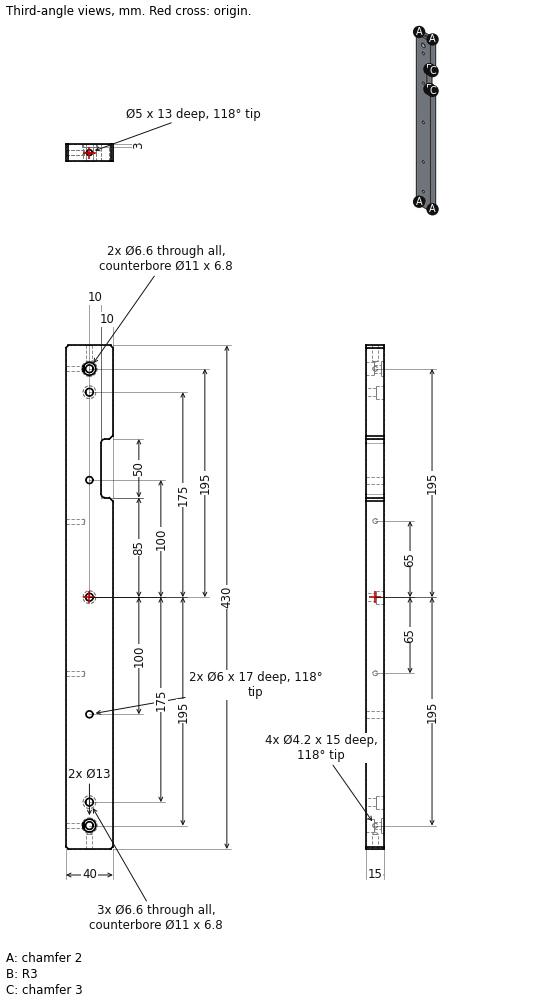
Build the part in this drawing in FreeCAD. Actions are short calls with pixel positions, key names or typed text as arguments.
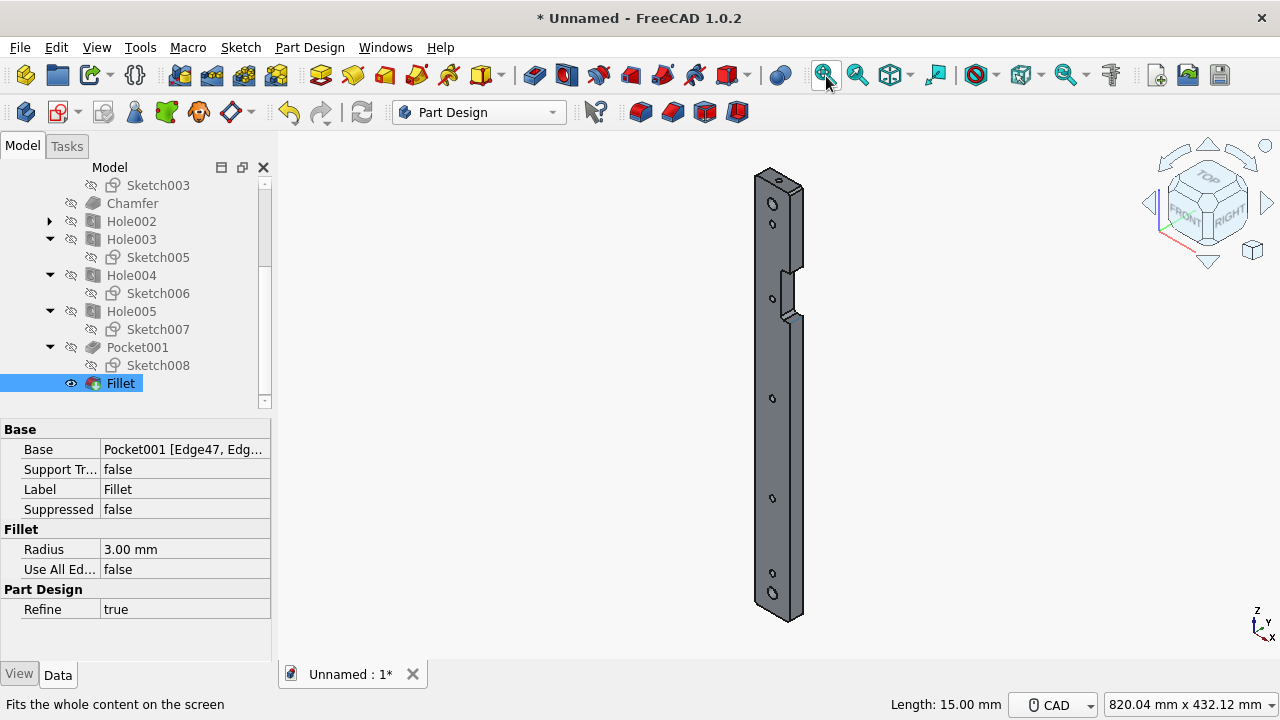
key(2)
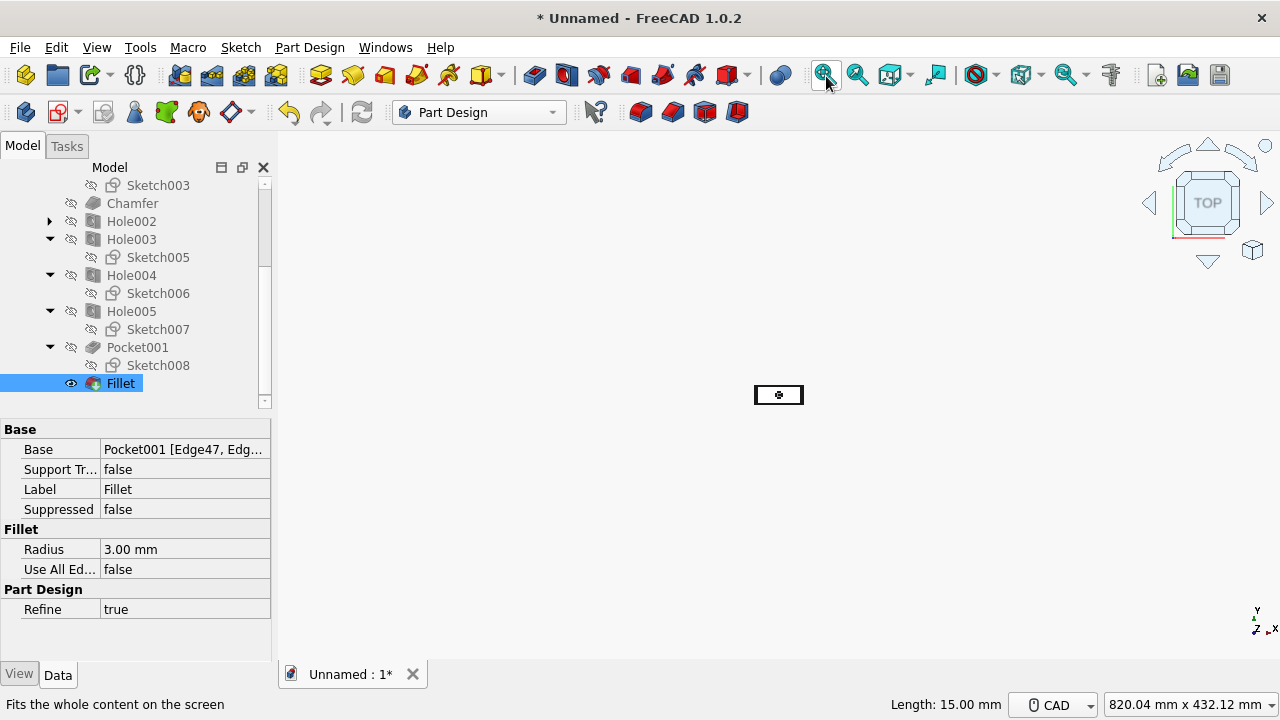
click(826, 76)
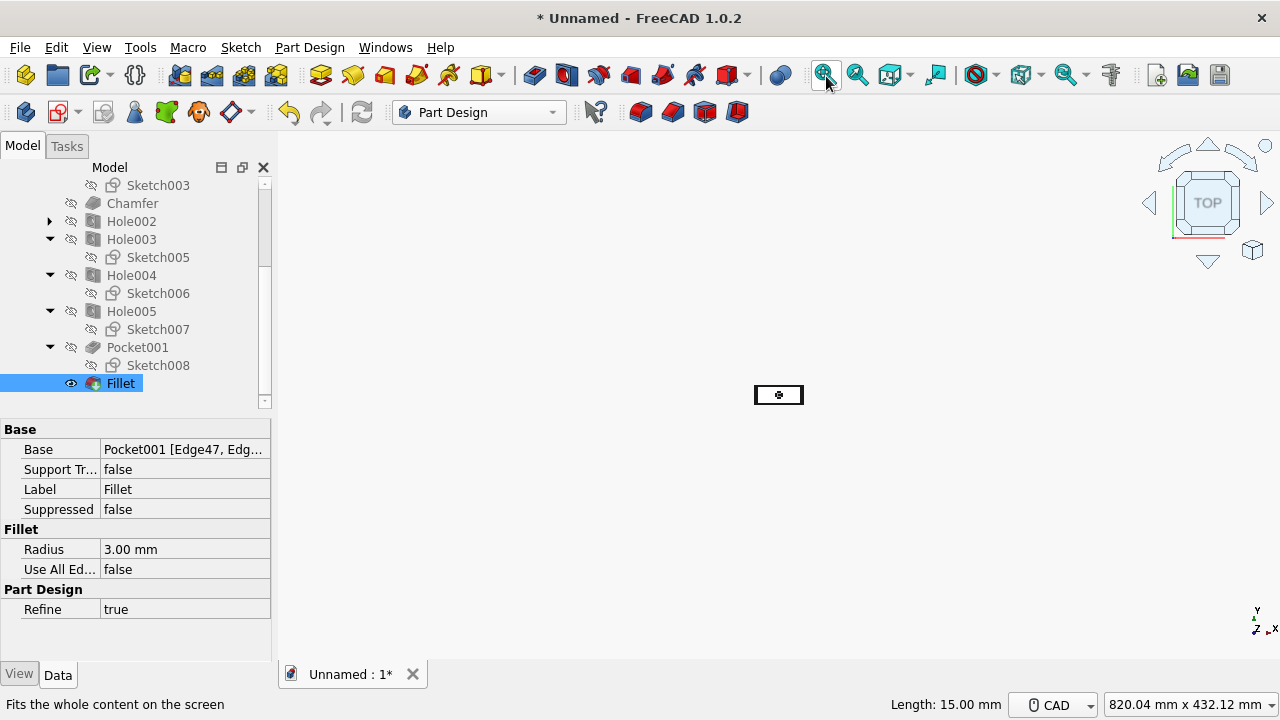
scroll(803, 394, up, 4)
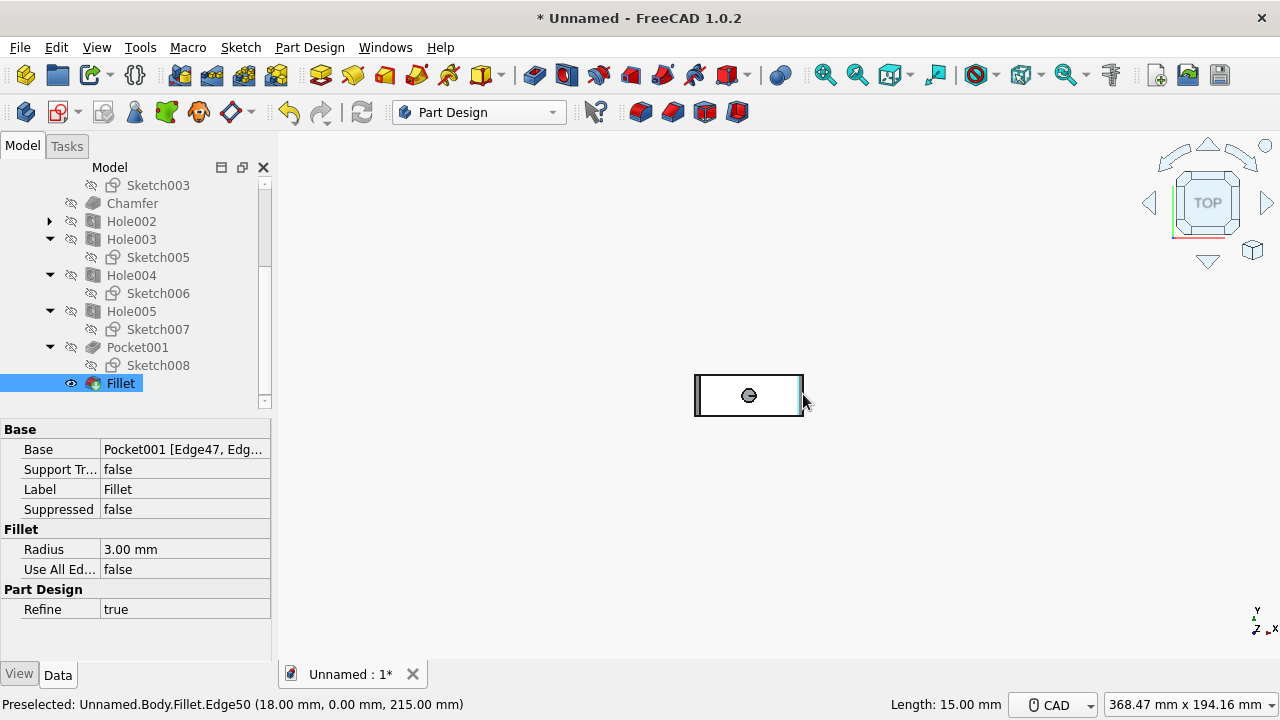
click(826, 76)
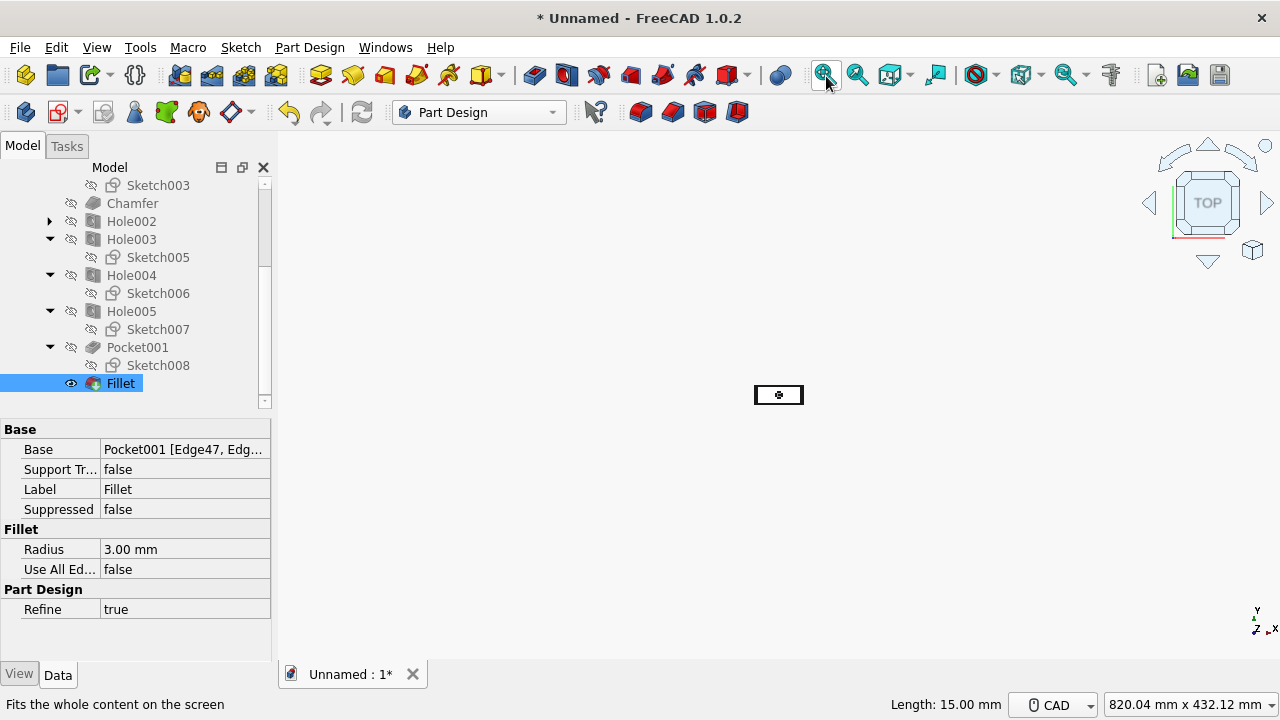
key(0)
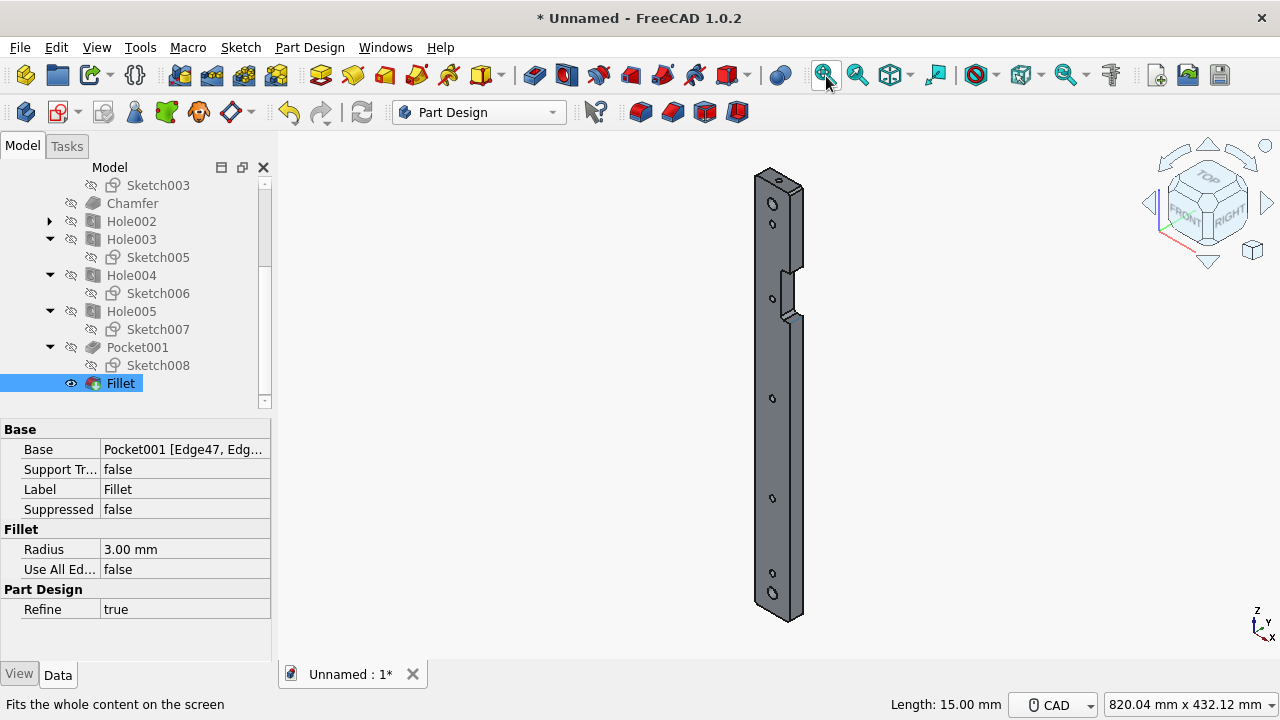
scroll(796, 269, up, 4)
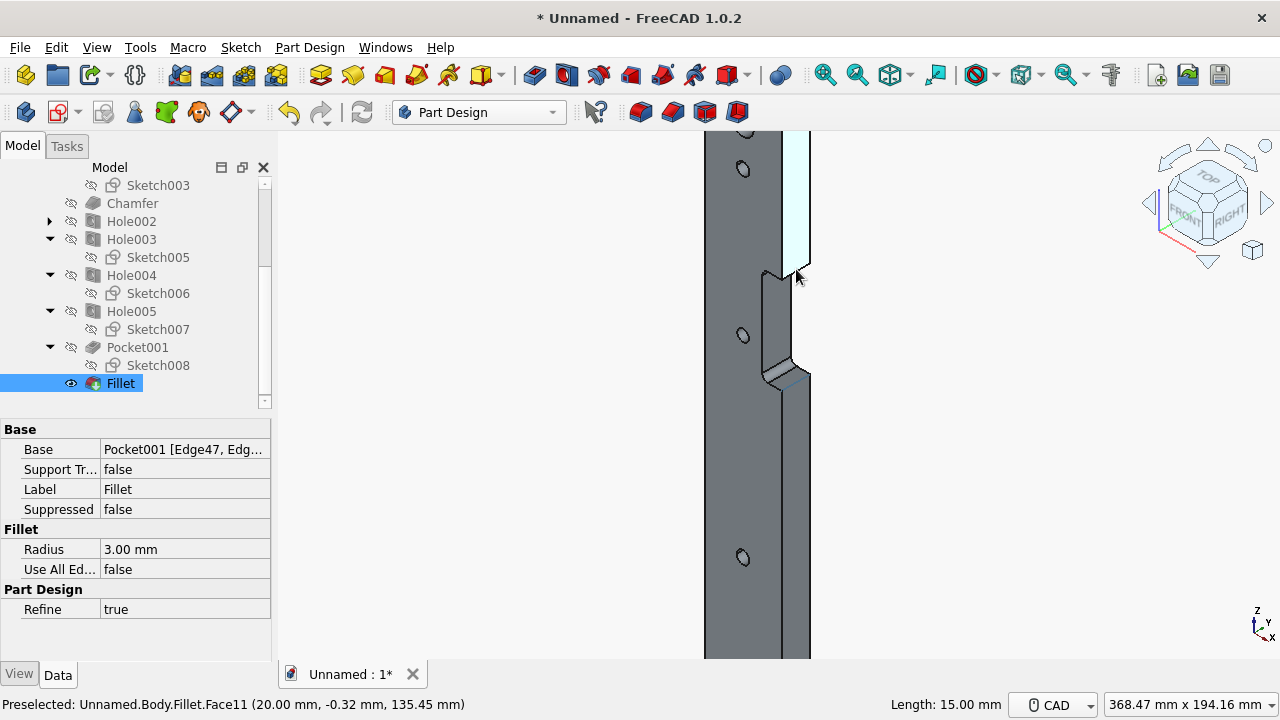
click(826, 76)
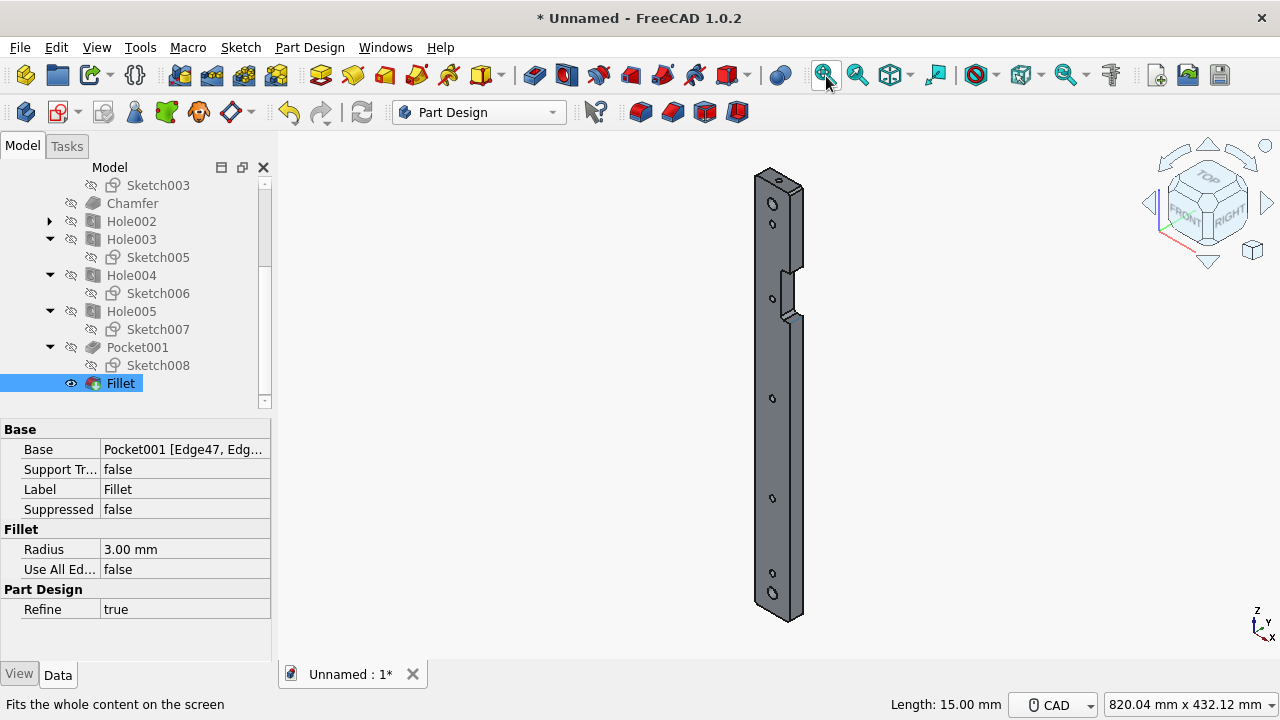
key(1)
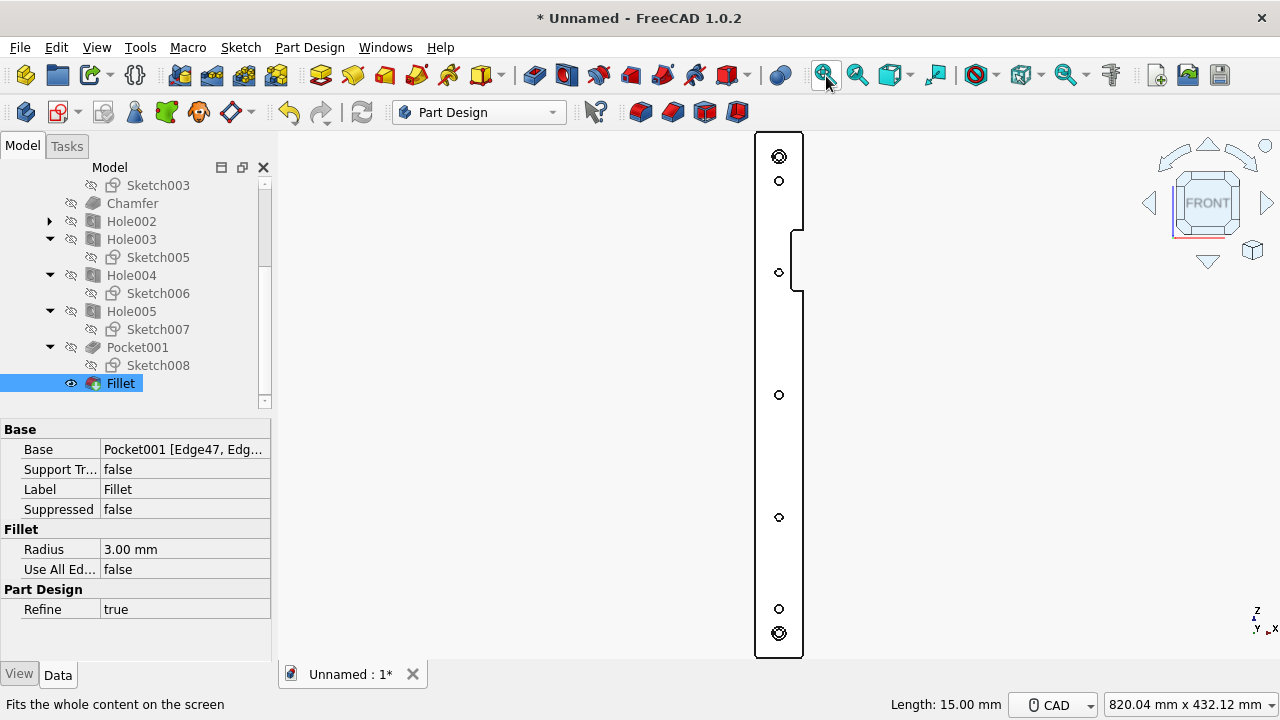
scroll(803, 229, up, 4)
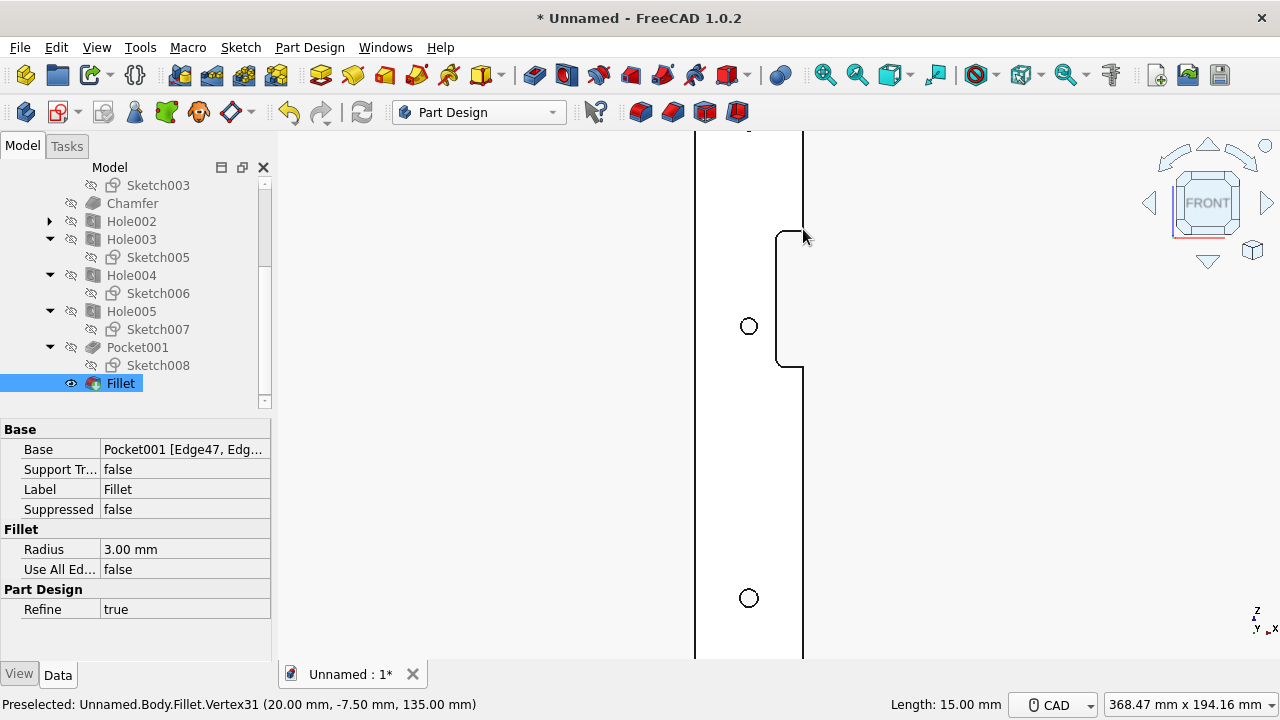
click(826, 76)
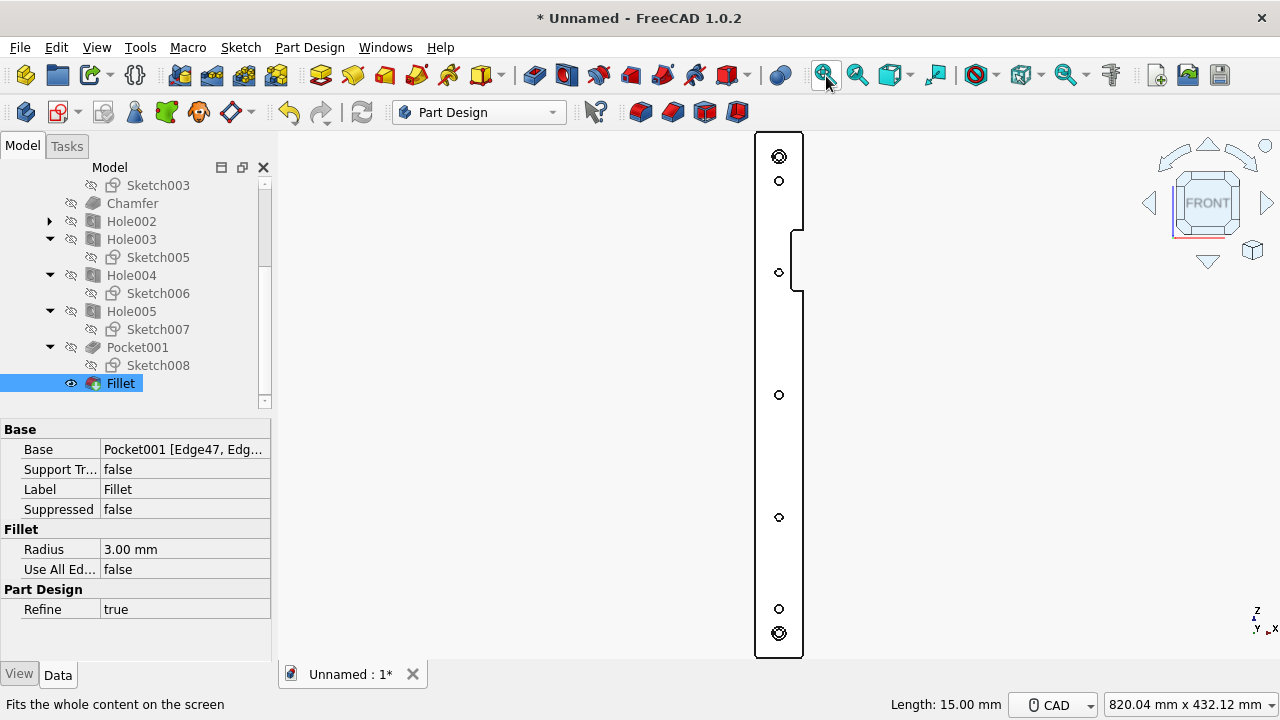
key(3)